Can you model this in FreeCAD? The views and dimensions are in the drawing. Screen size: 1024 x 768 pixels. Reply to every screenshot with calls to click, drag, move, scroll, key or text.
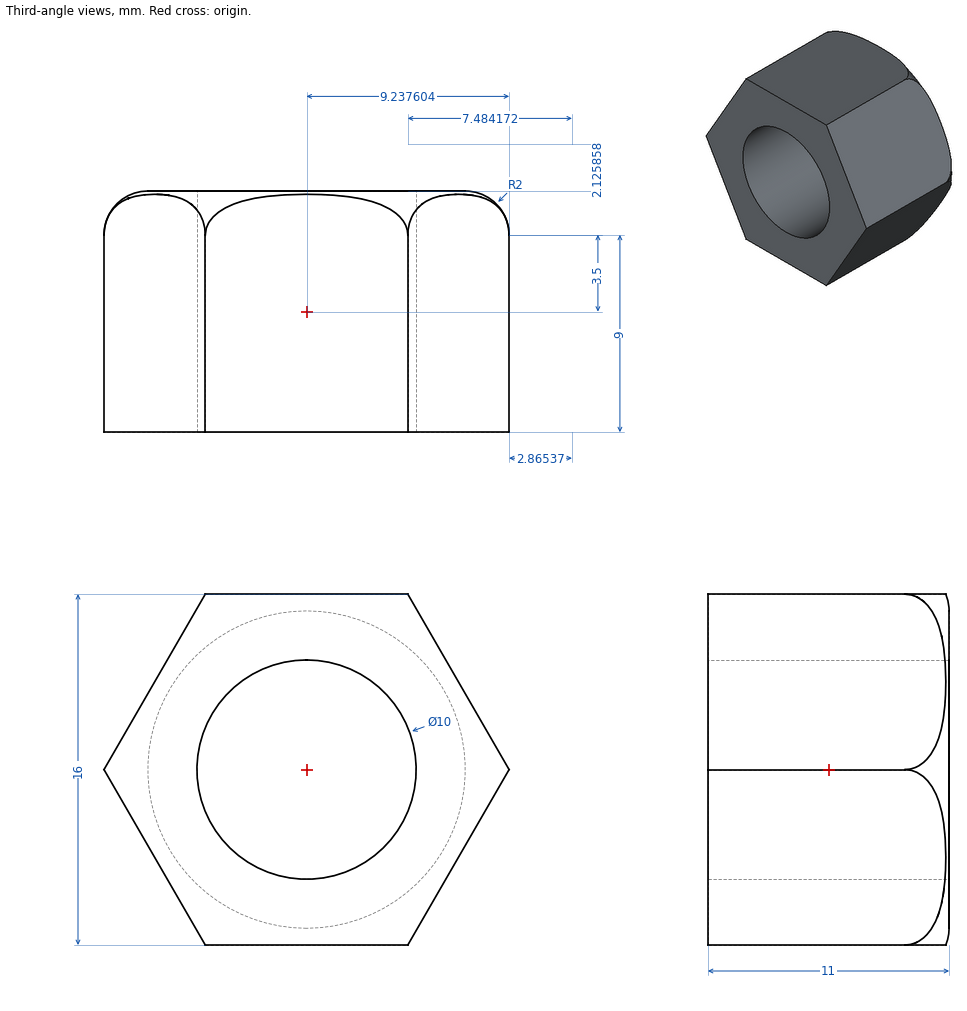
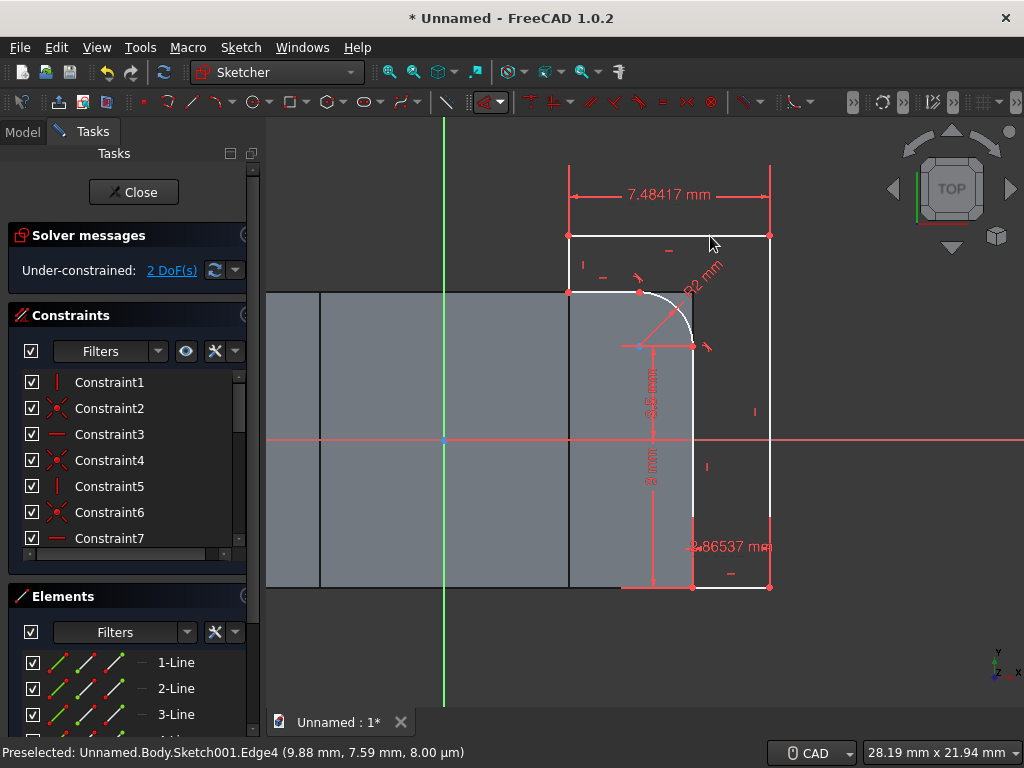
click(569, 253)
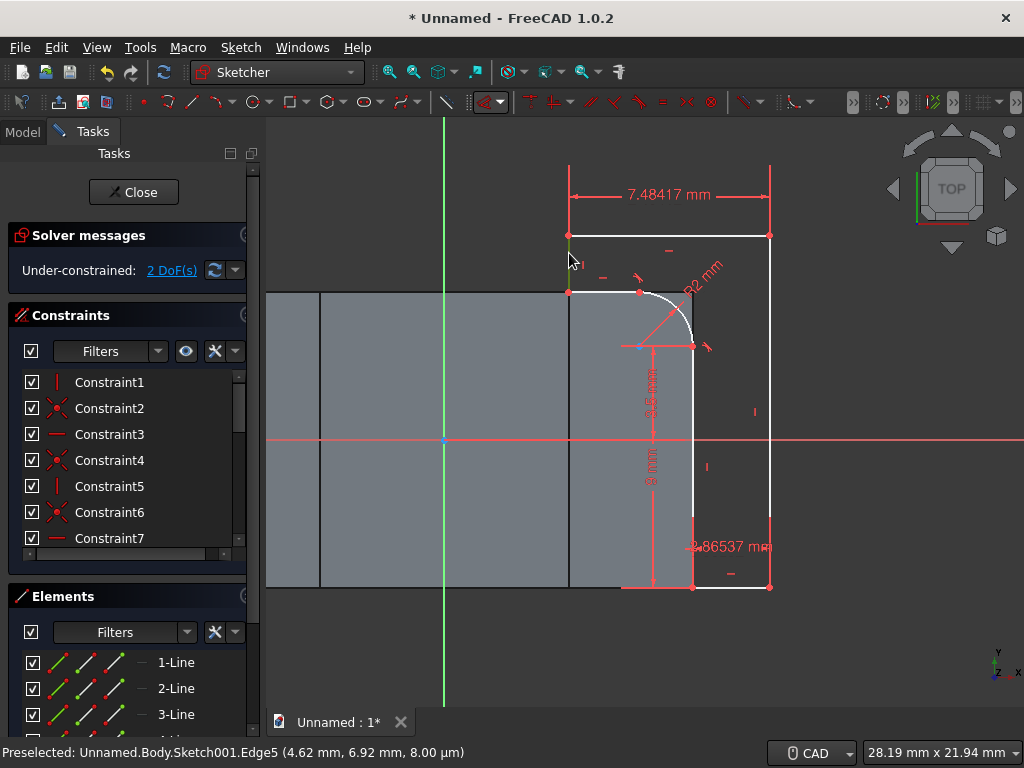
key(i)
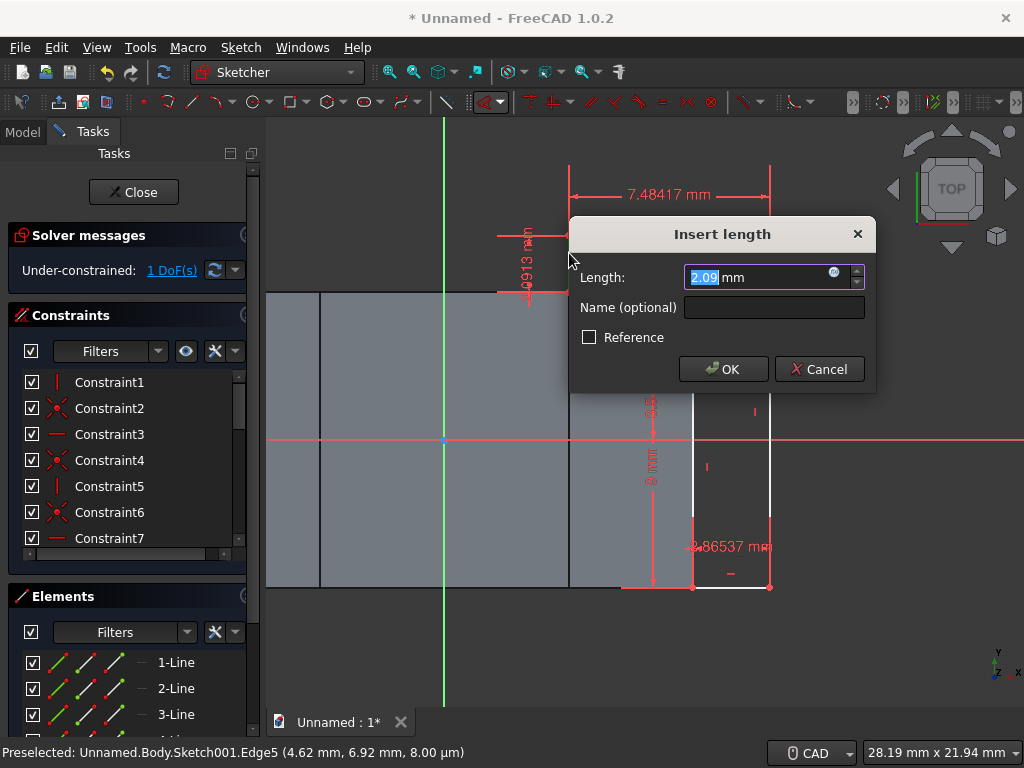
text(2.125858)
key(Return)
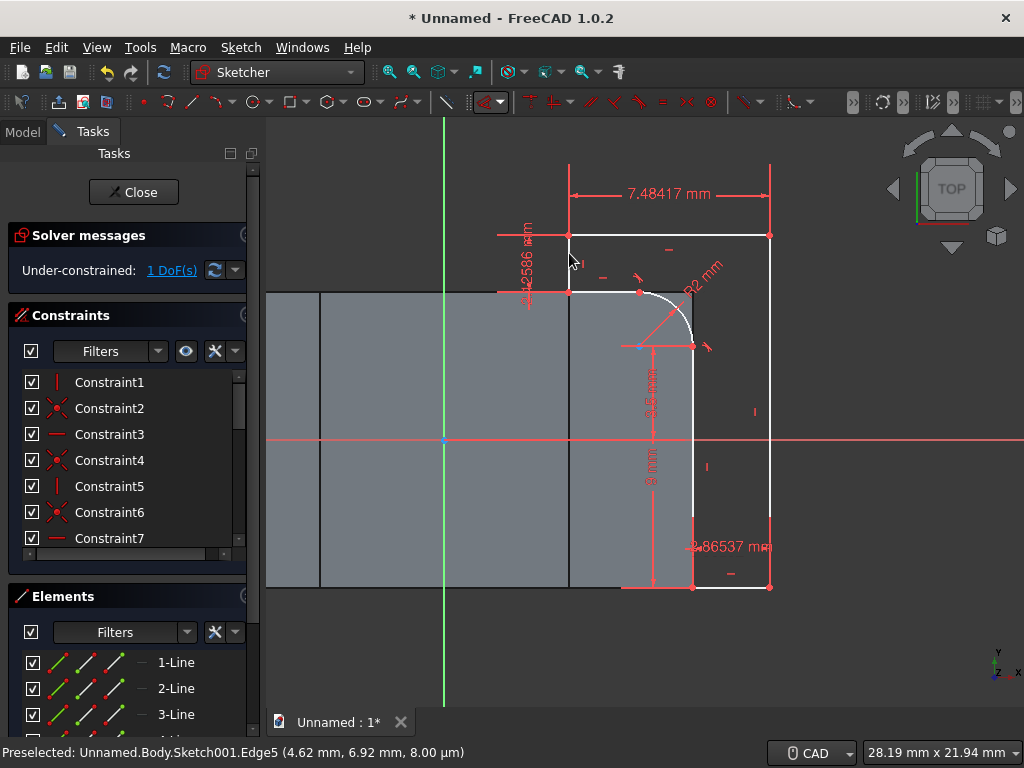
click(693, 346)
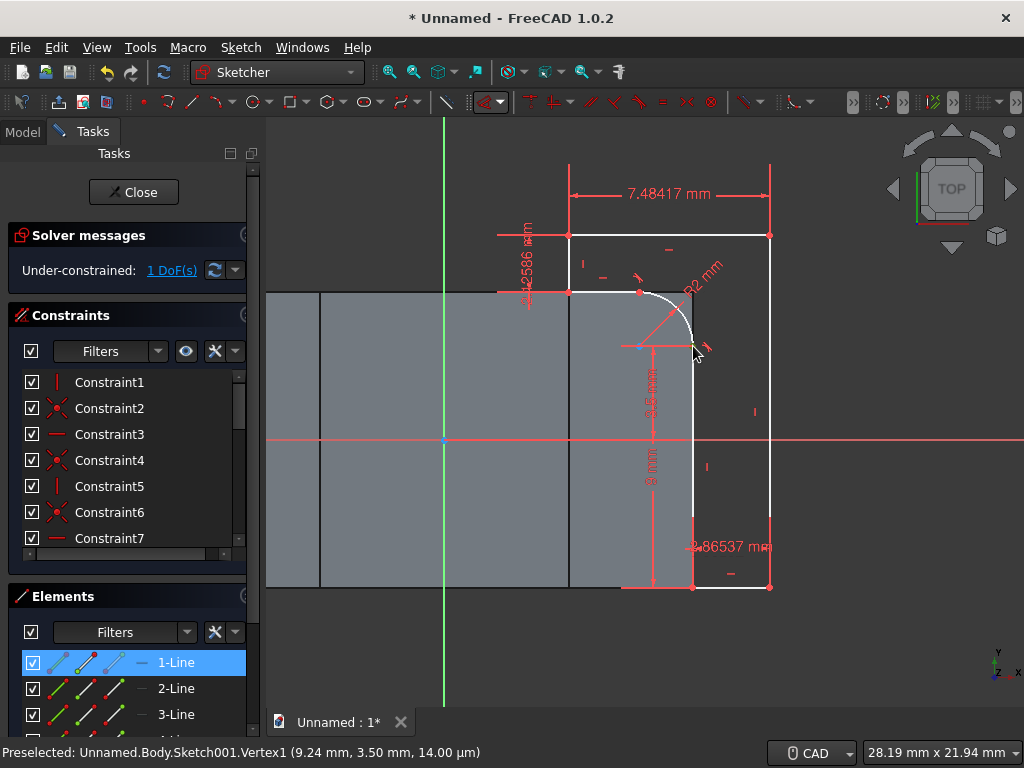
key(l)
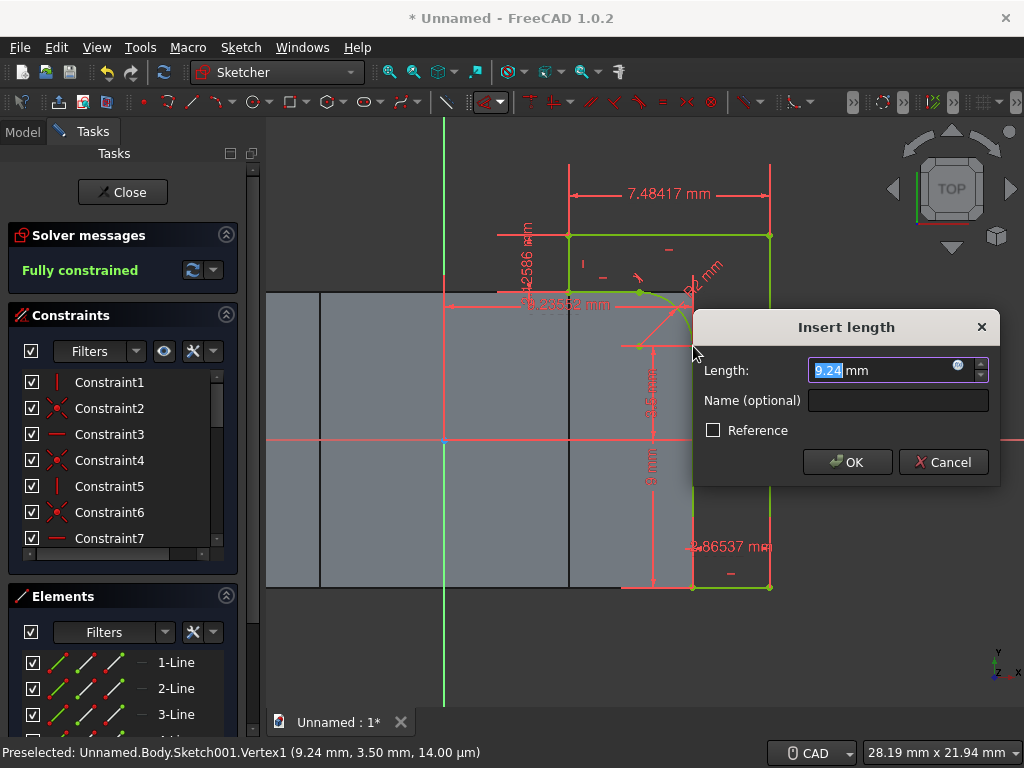
text(9.237604)
key(Return)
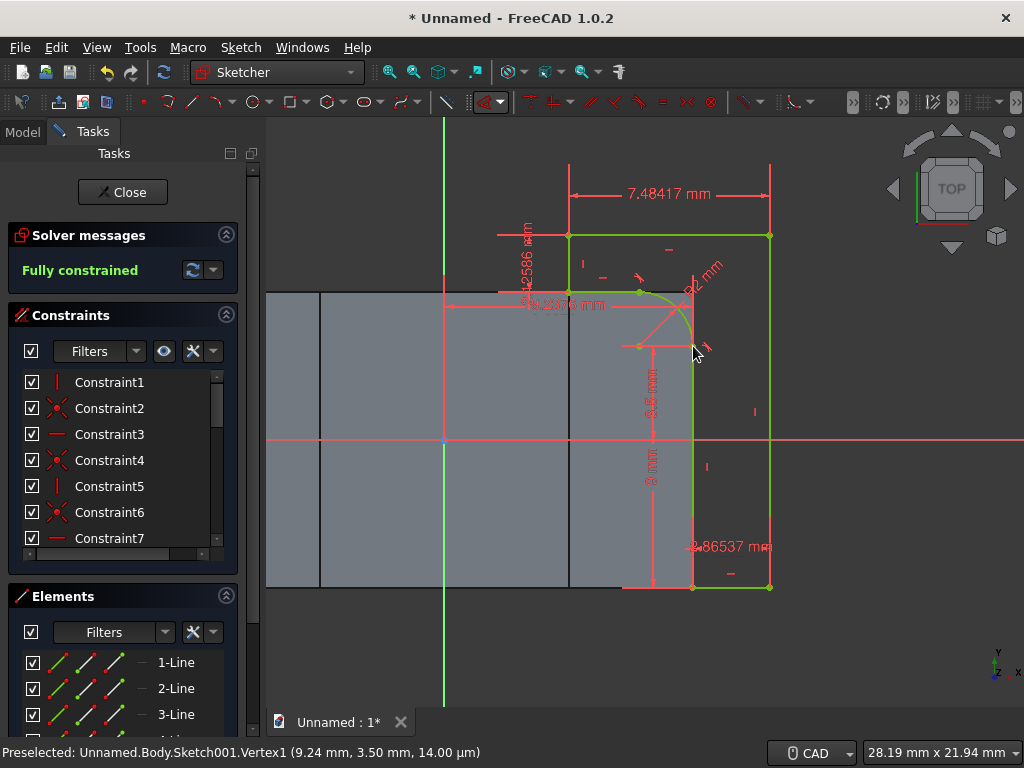
click(123, 192)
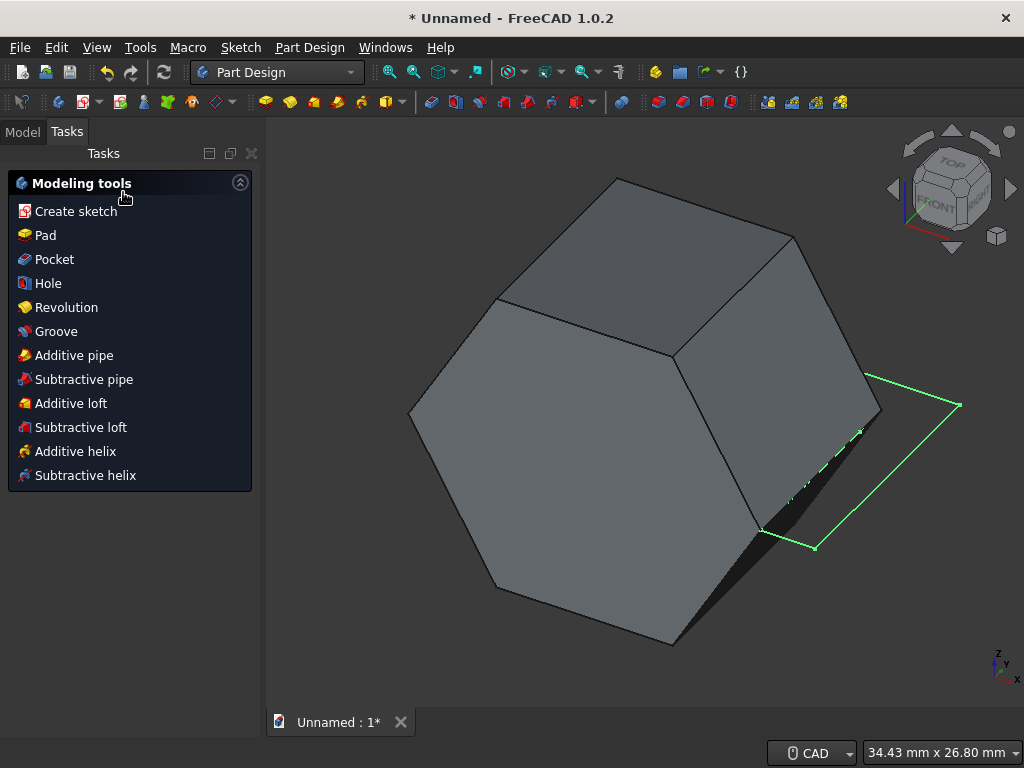
click(480, 102)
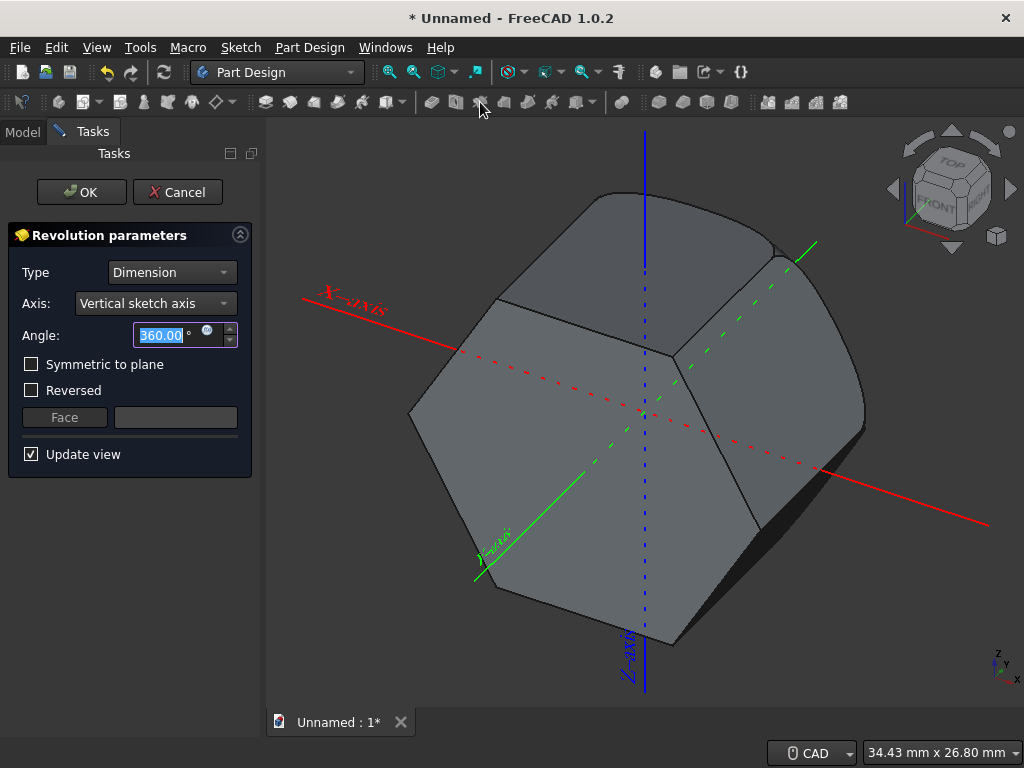
click(82, 192)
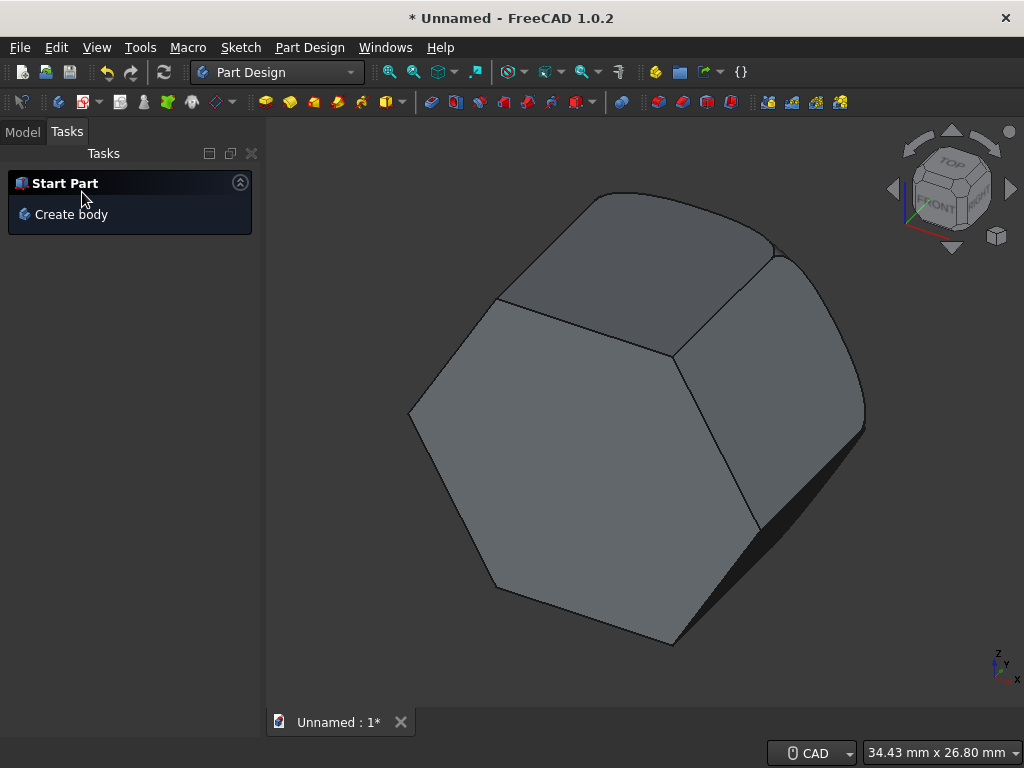
key(4)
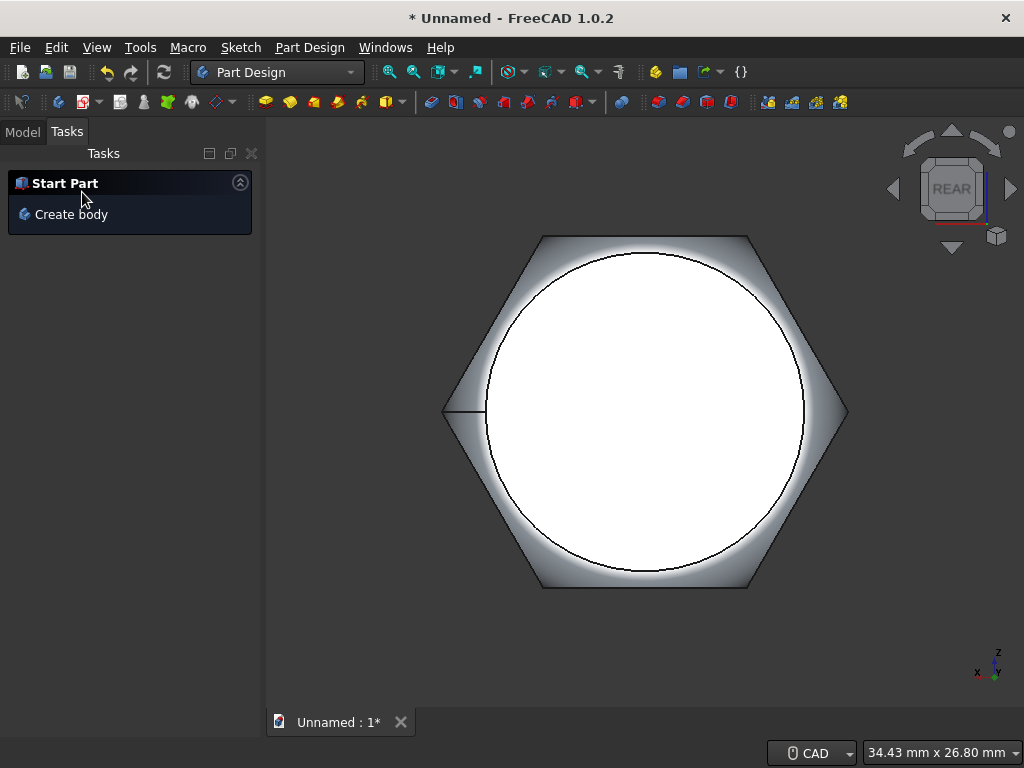
click(645, 411)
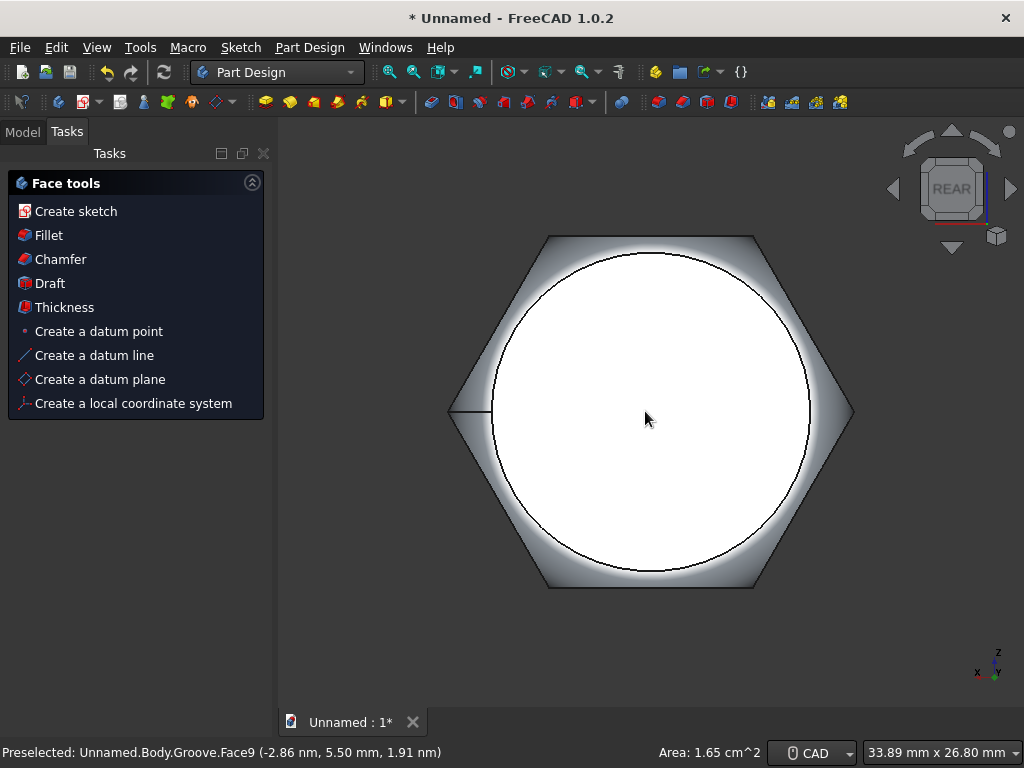
click(84, 102)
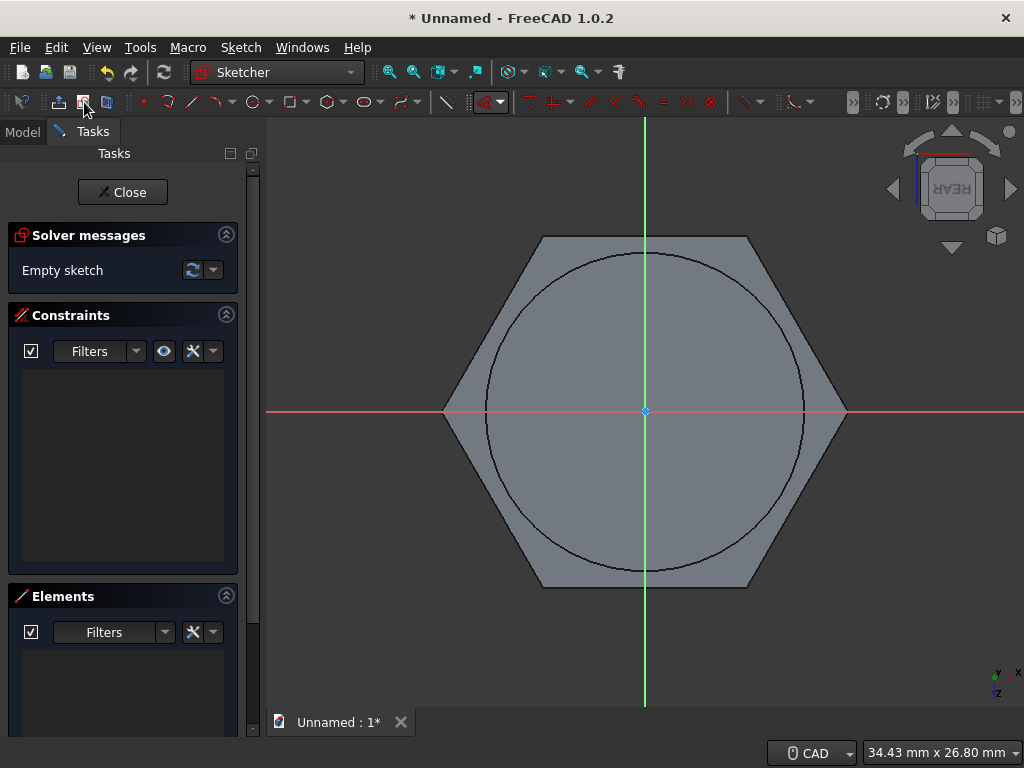
scroll(728, 412, up, 3)